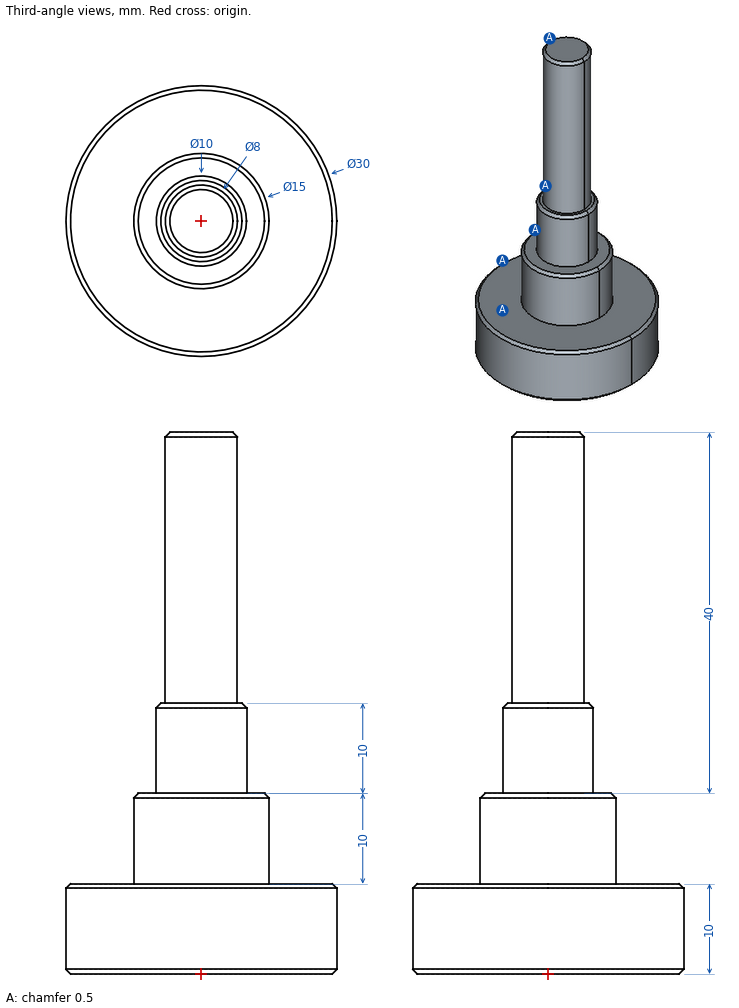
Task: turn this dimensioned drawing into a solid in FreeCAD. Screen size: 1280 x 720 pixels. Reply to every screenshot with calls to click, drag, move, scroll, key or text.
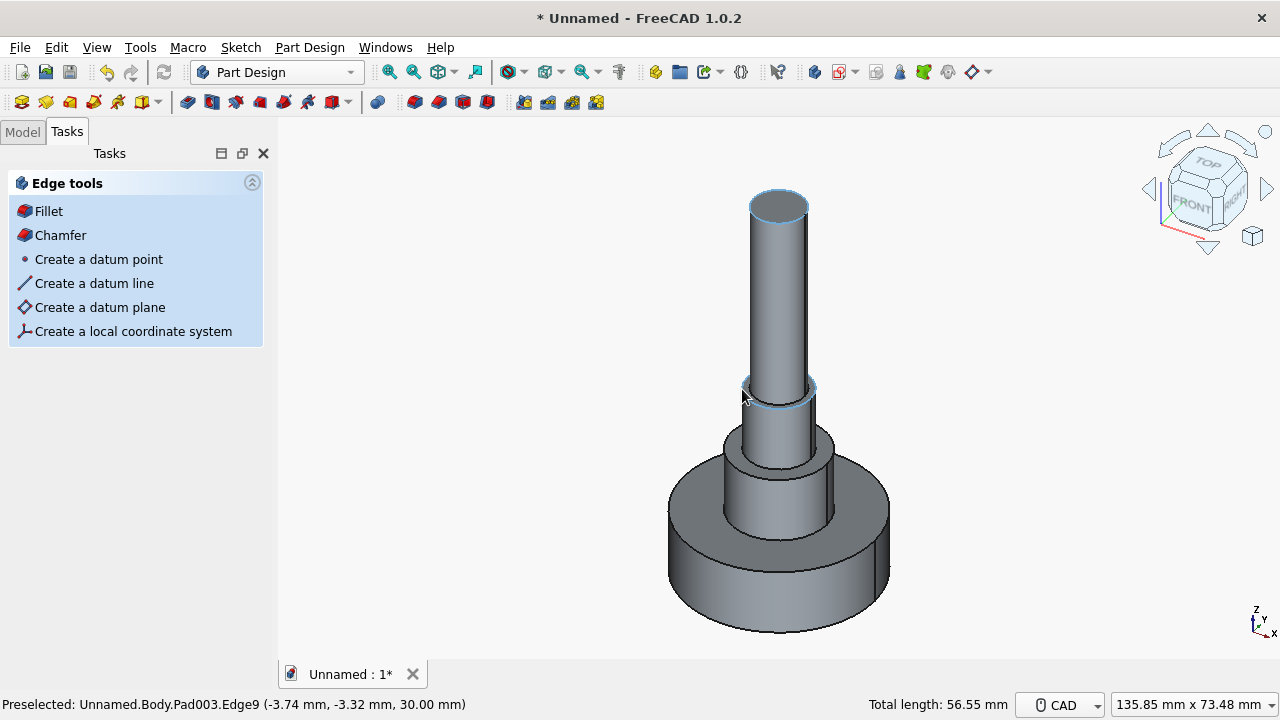
click(669, 514, ctrl)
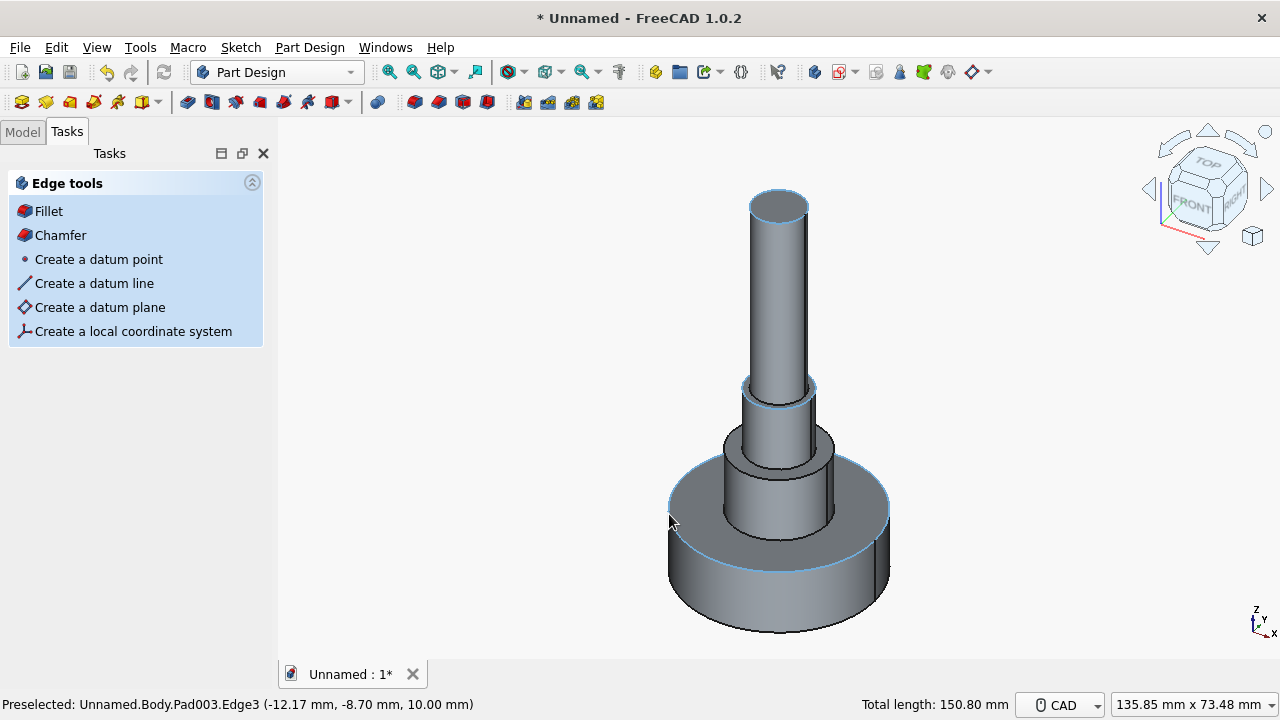
click(724, 451, ctrl)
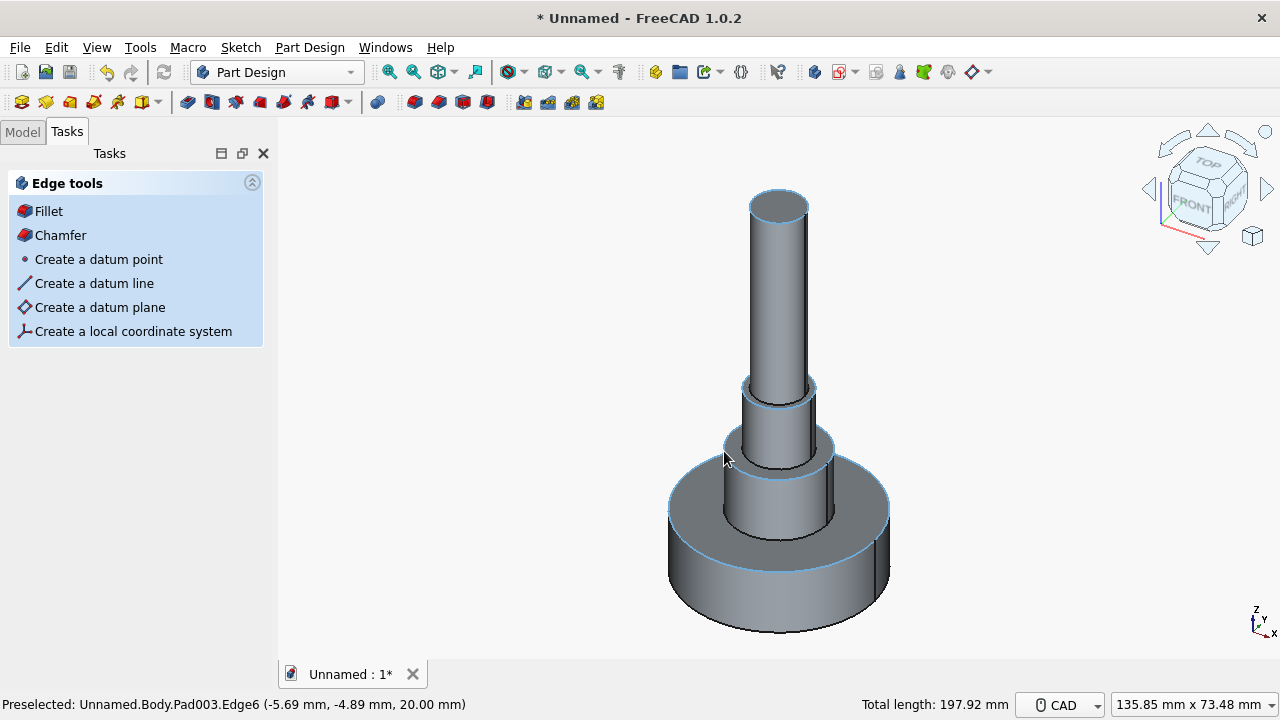
key(0)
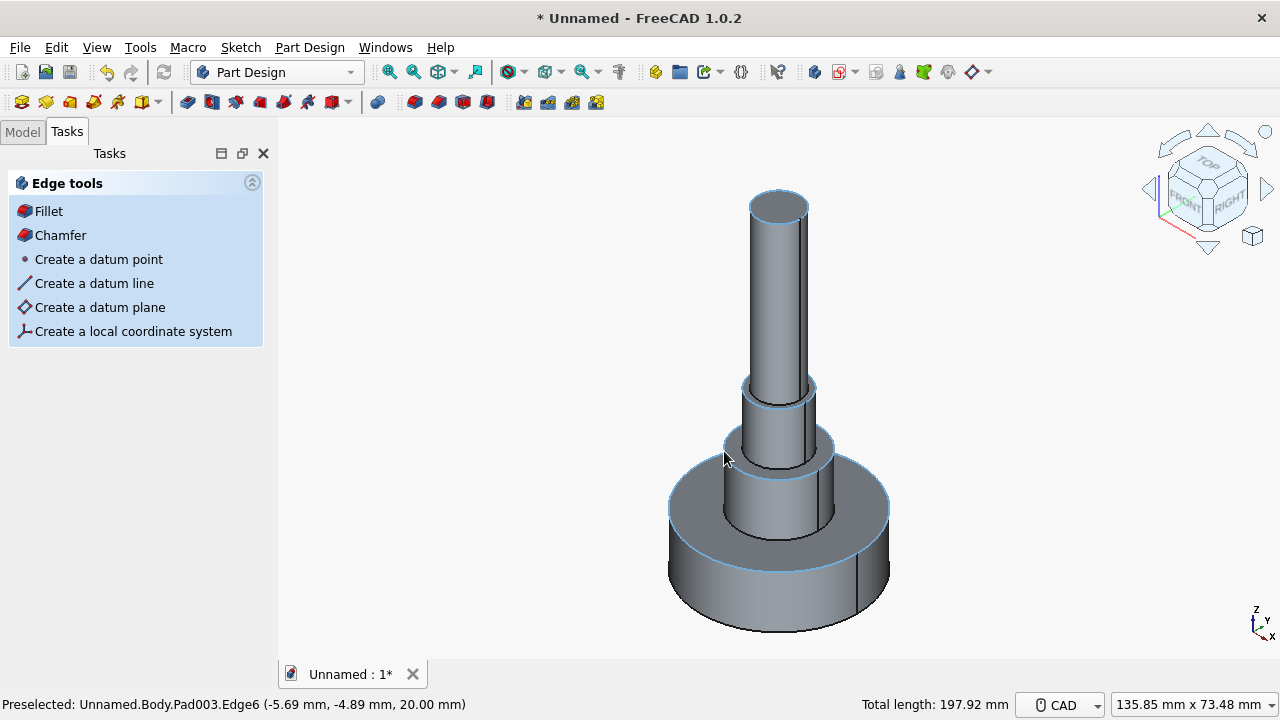
click(390, 72)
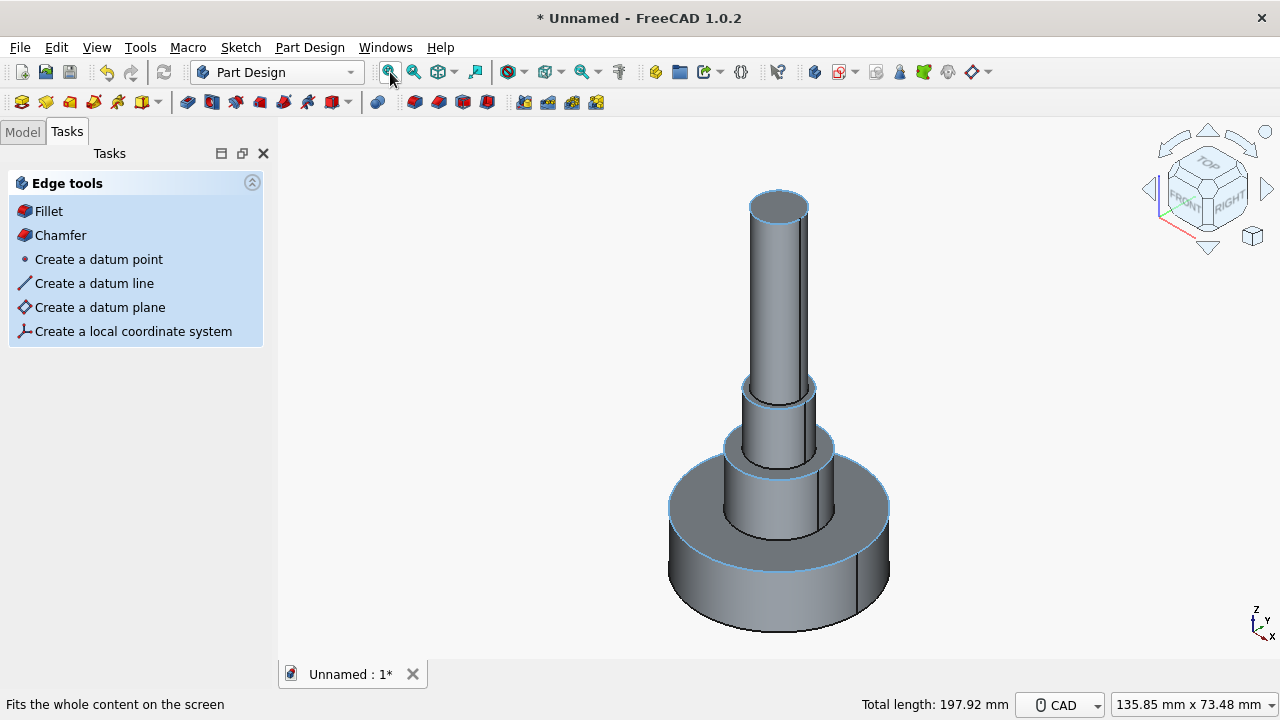
click(680, 597, ctrl)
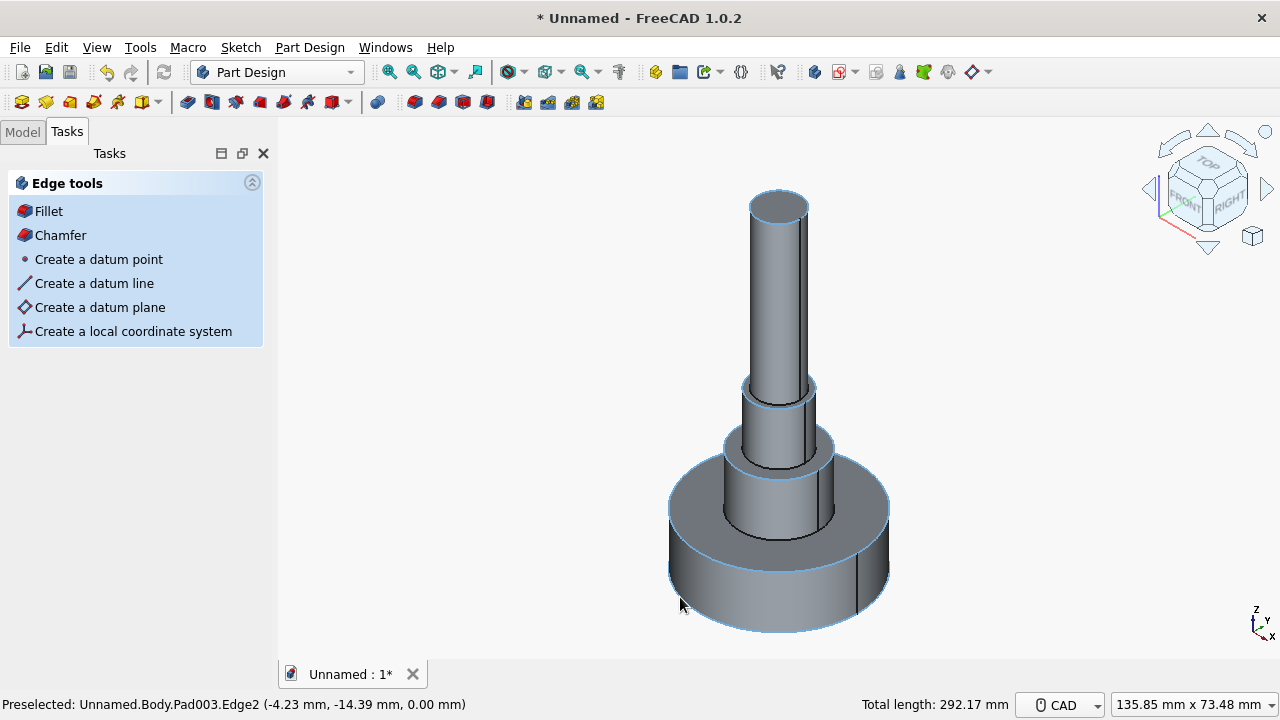
click(440, 102)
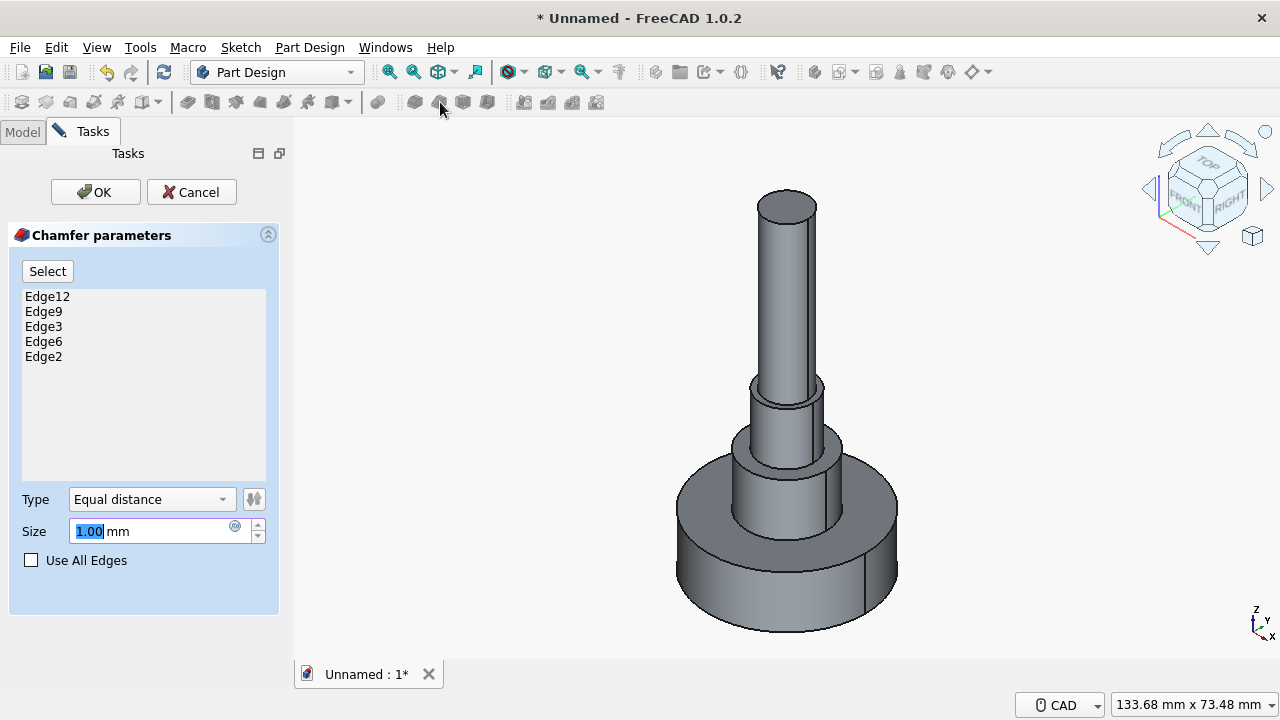
text(0.5)
key(Tab)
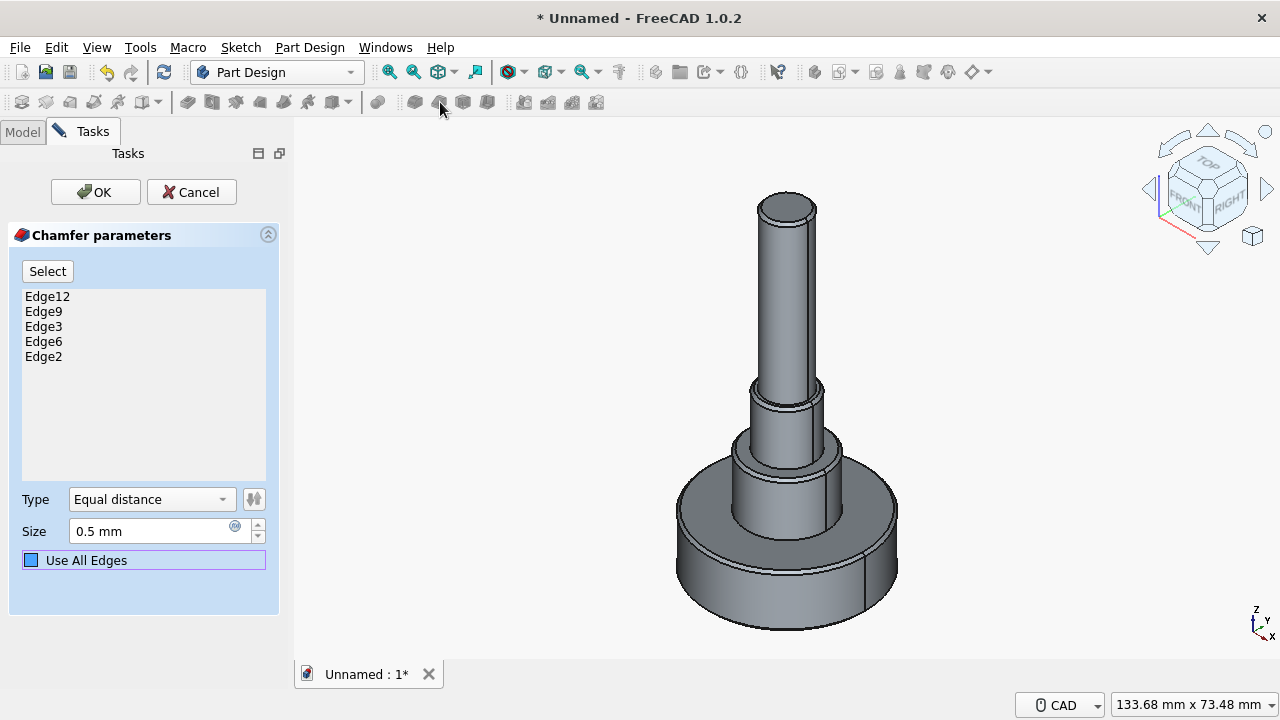
click(96, 192)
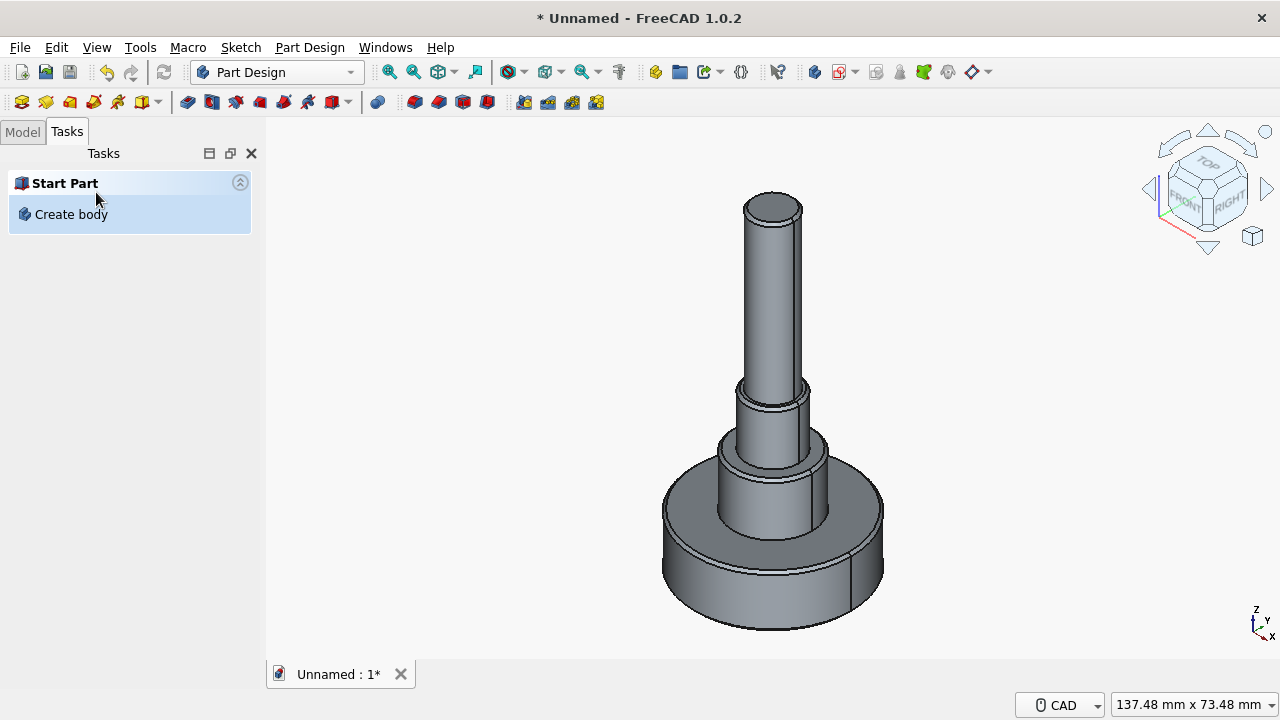
click(390, 72)